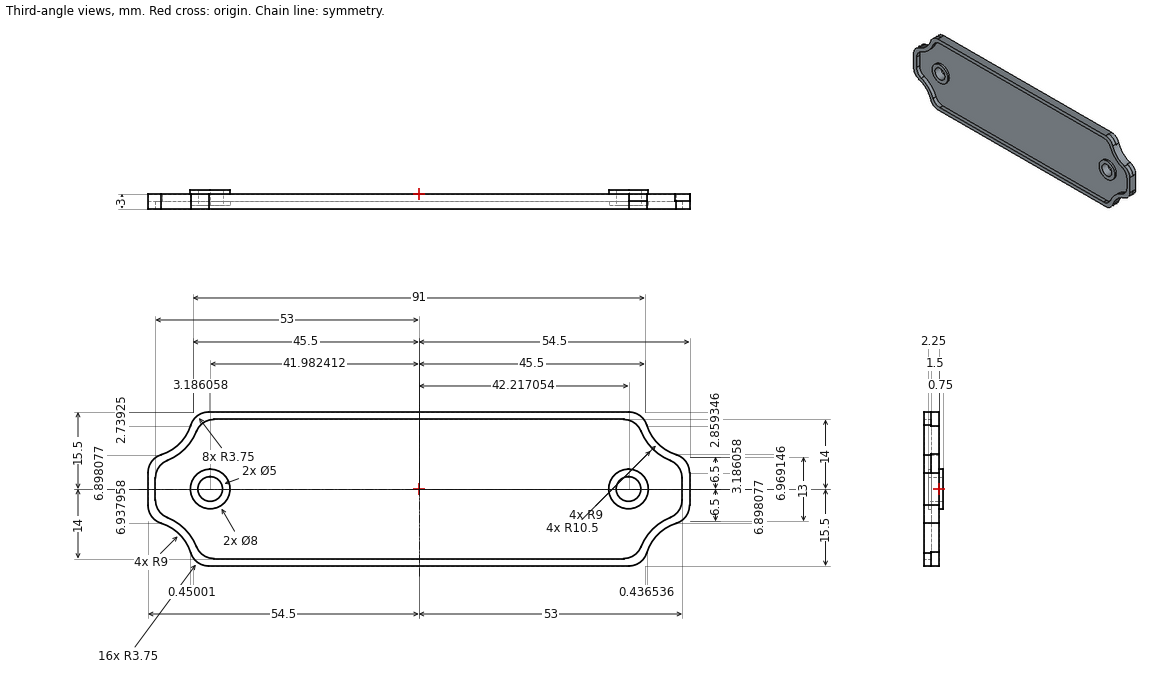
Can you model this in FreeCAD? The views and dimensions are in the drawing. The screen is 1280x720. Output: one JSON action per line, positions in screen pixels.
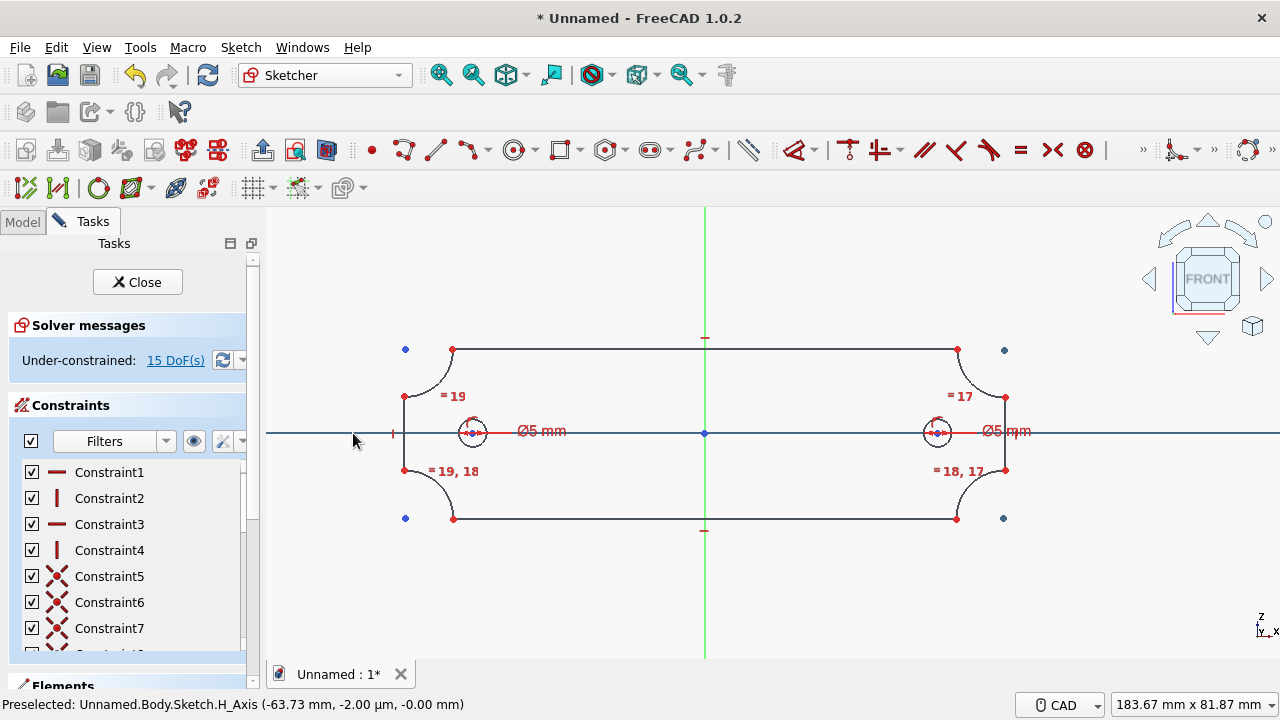
{"action": "left_click", "coordinate": [1054, 150]}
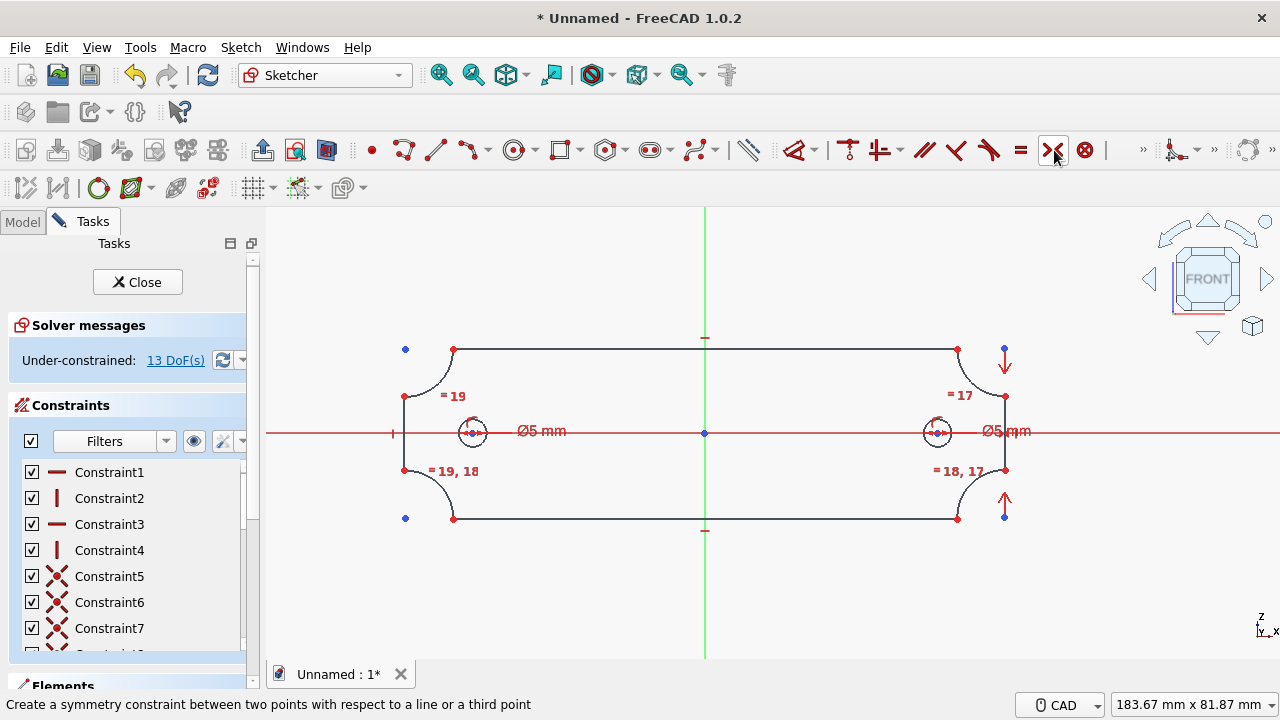
{"action": "left_click", "coordinate": [1005, 517]}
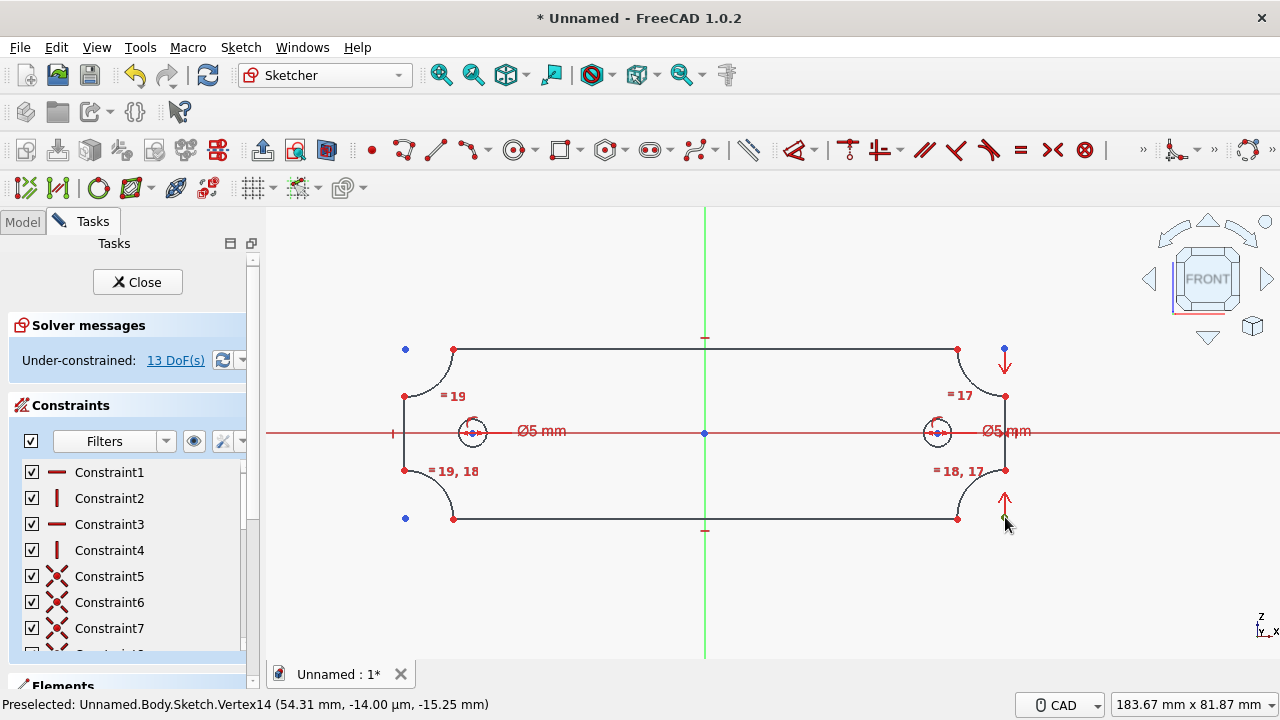
{"action": "left_click", "coordinate": [406, 518]}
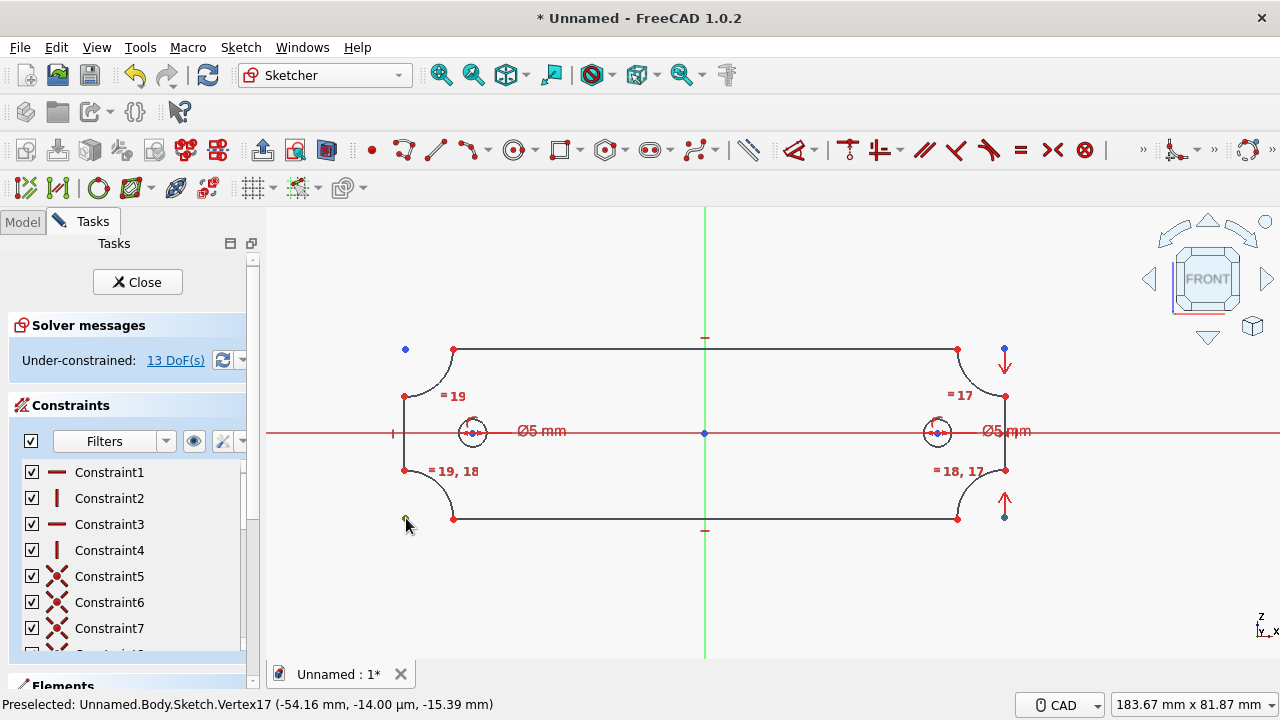
{"action": "left_click", "coordinate": [705, 603]}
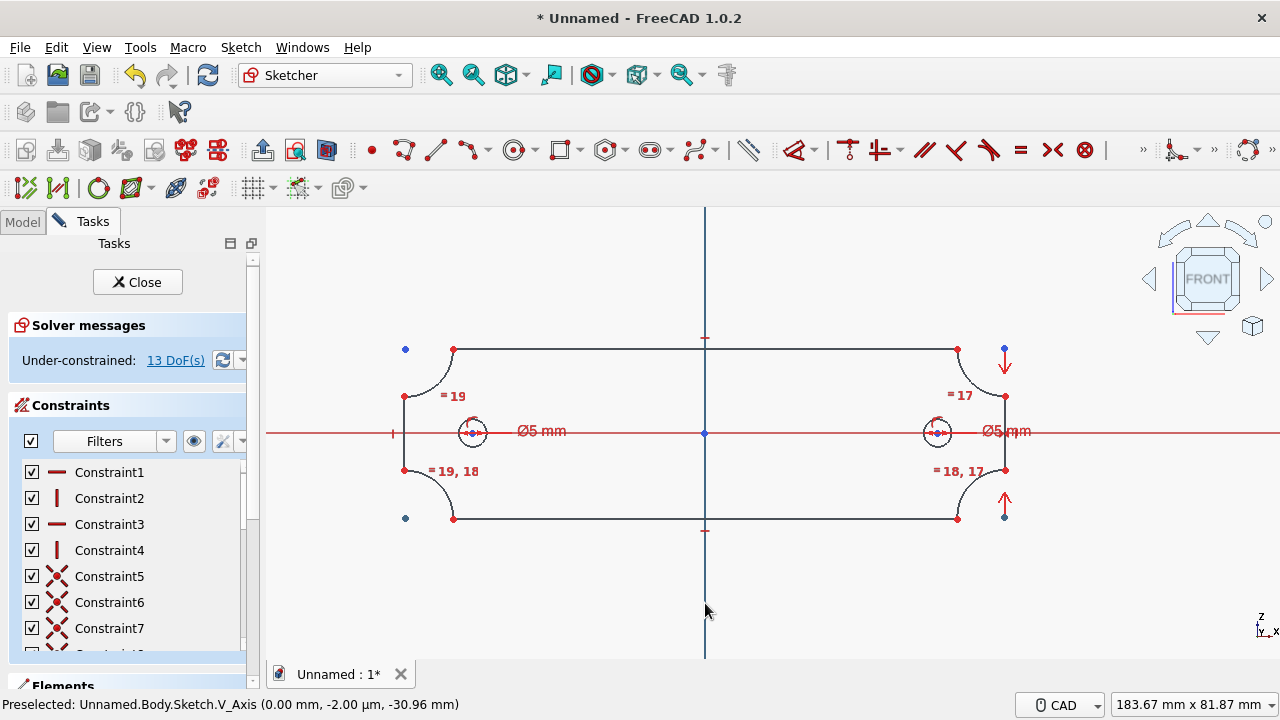
{"action": "left_click", "coordinate": [1054, 150]}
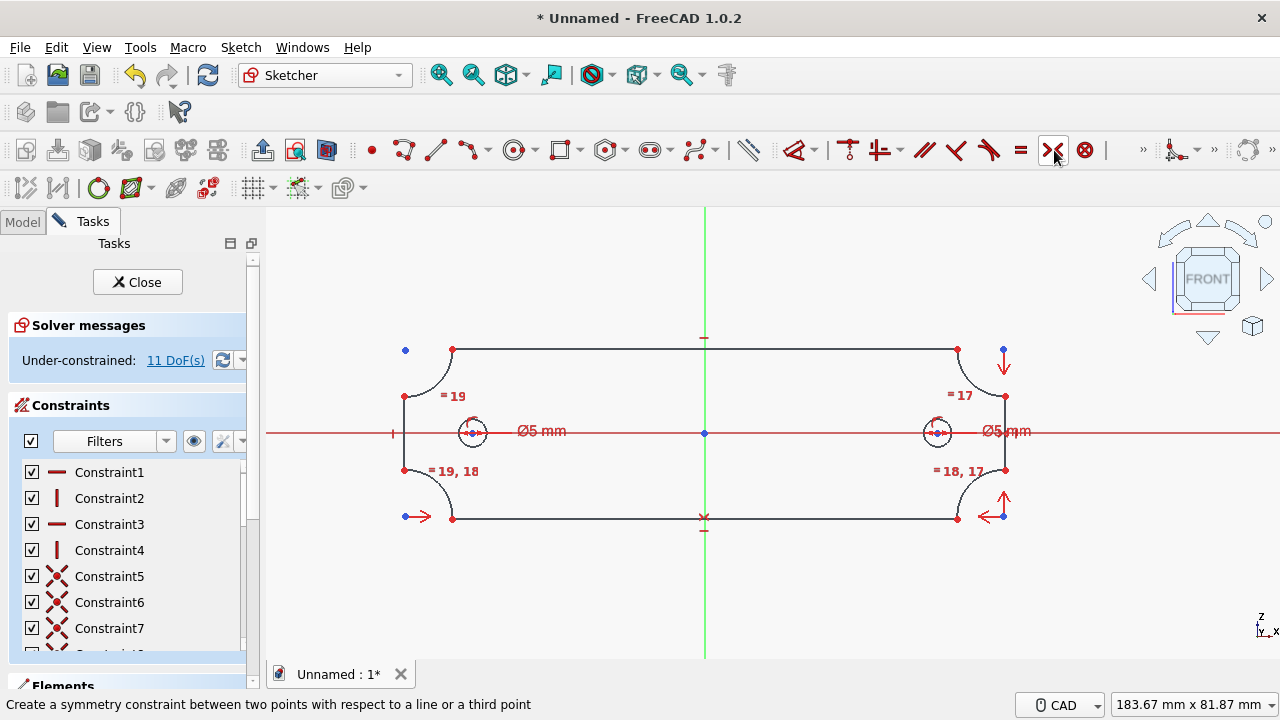
{"action": "left_click", "coordinate": [1004, 350]}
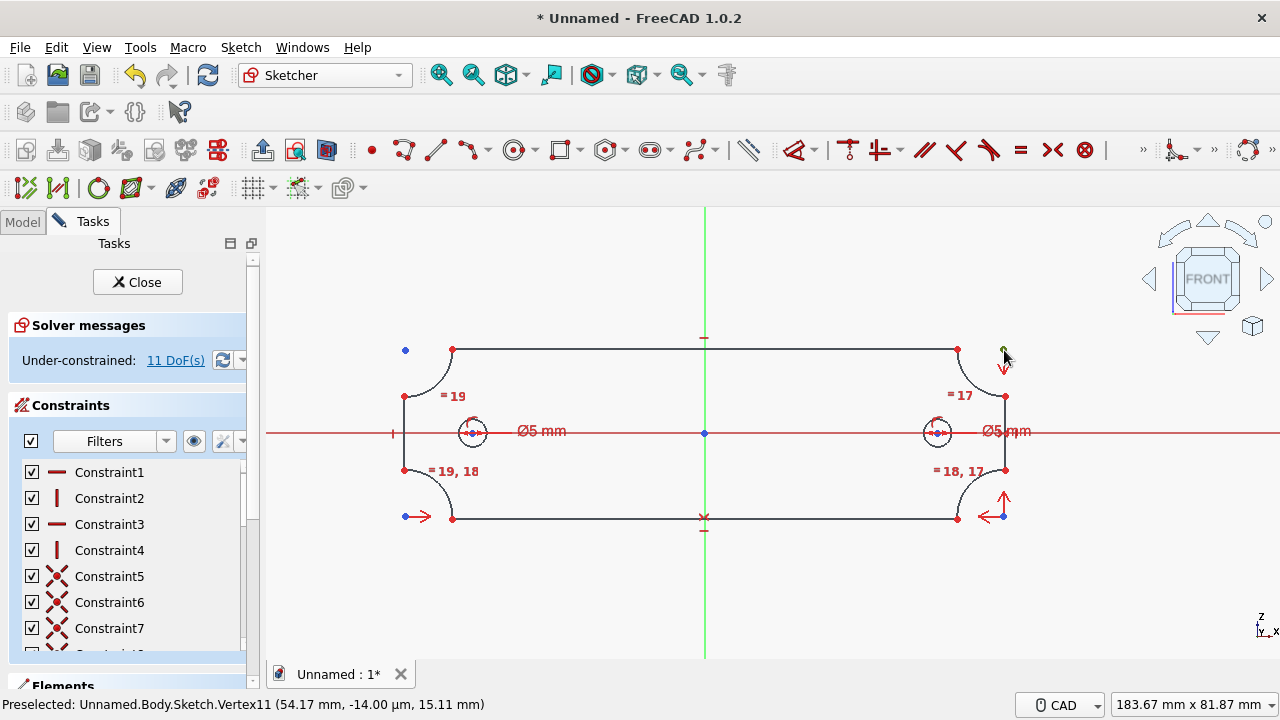
{"action": "left_click", "coordinate": [406, 350]}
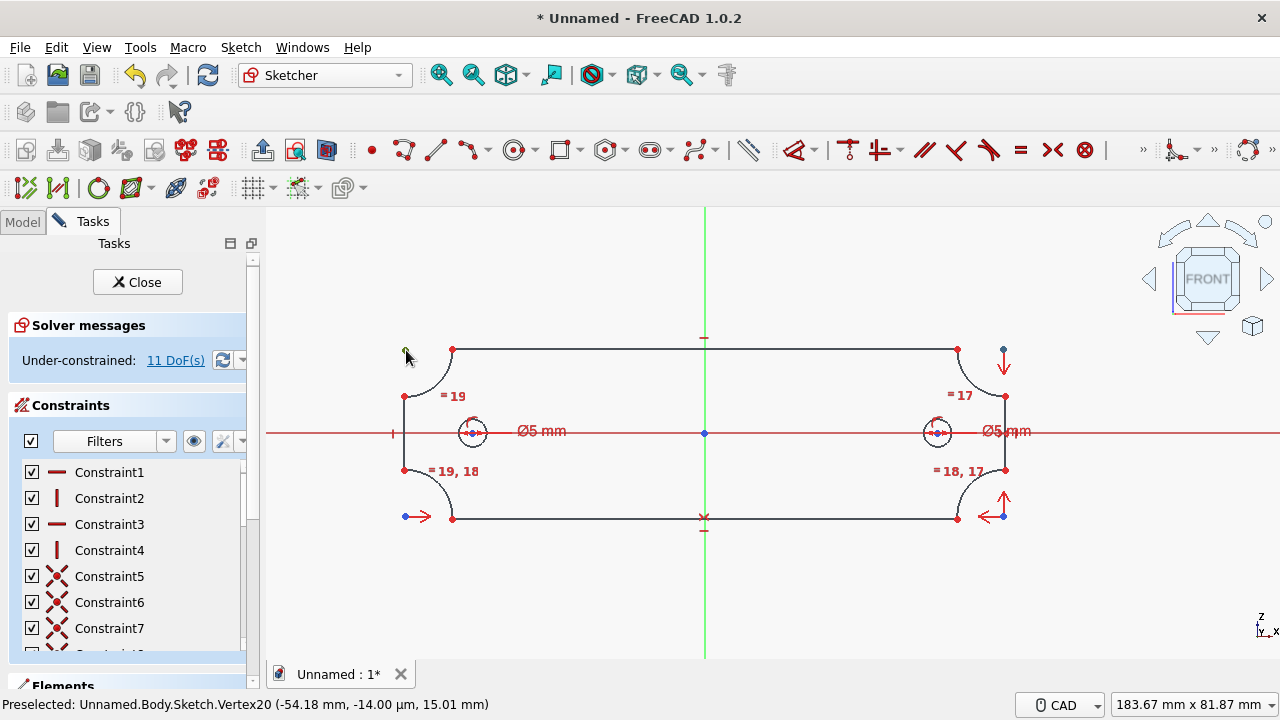
{"action": "left_click", "coordinate": [705, 603]}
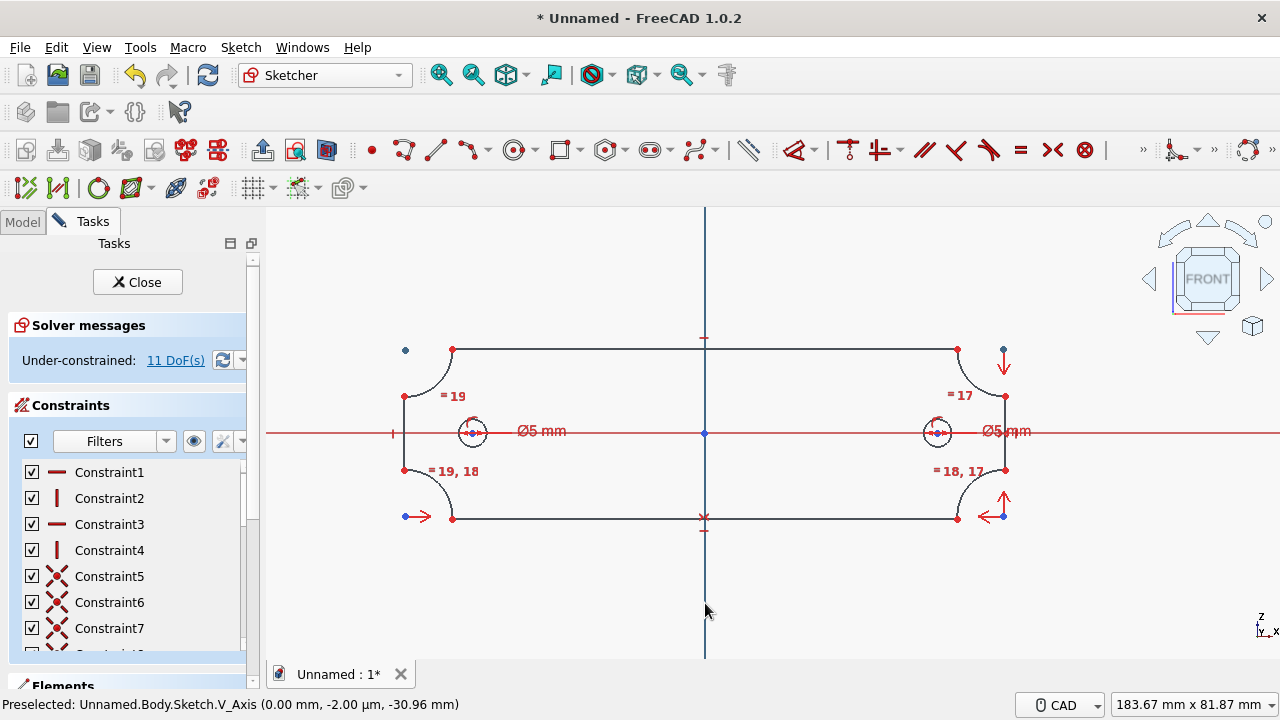
{"action": "left_click", "coordinate": [1054, 150]}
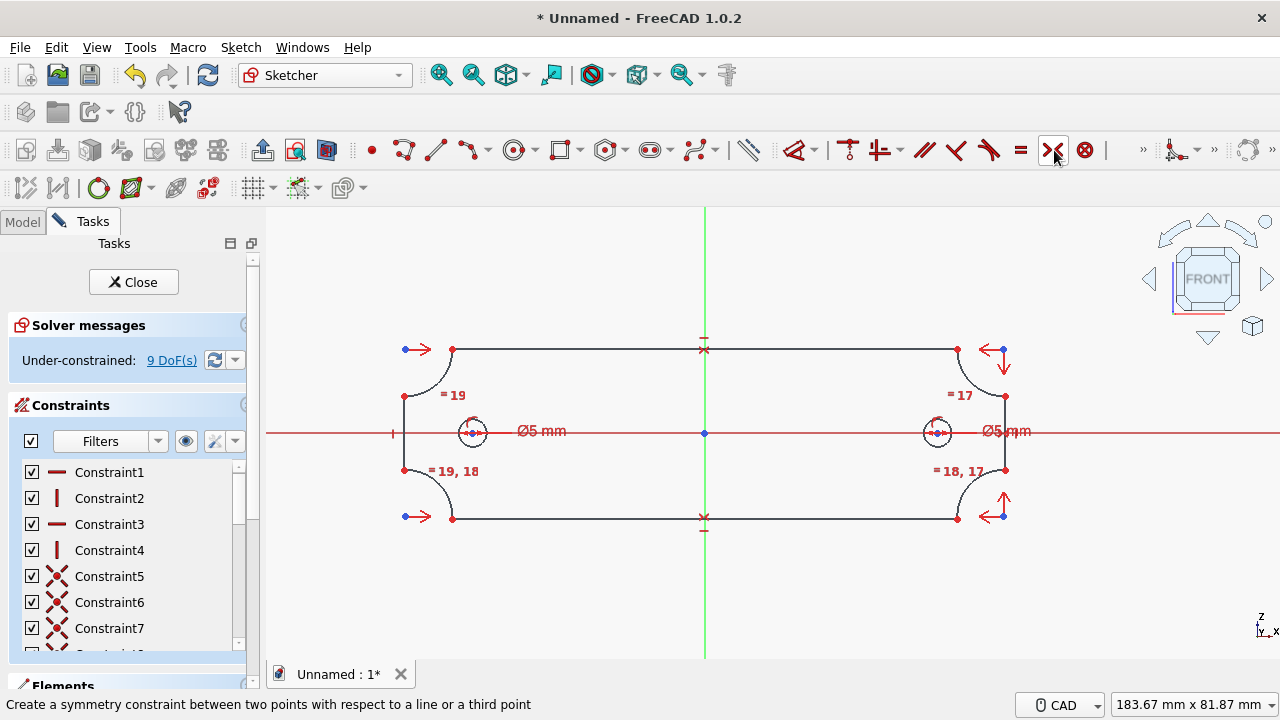
{"action": "left_click", "coordinate": [794, 150]}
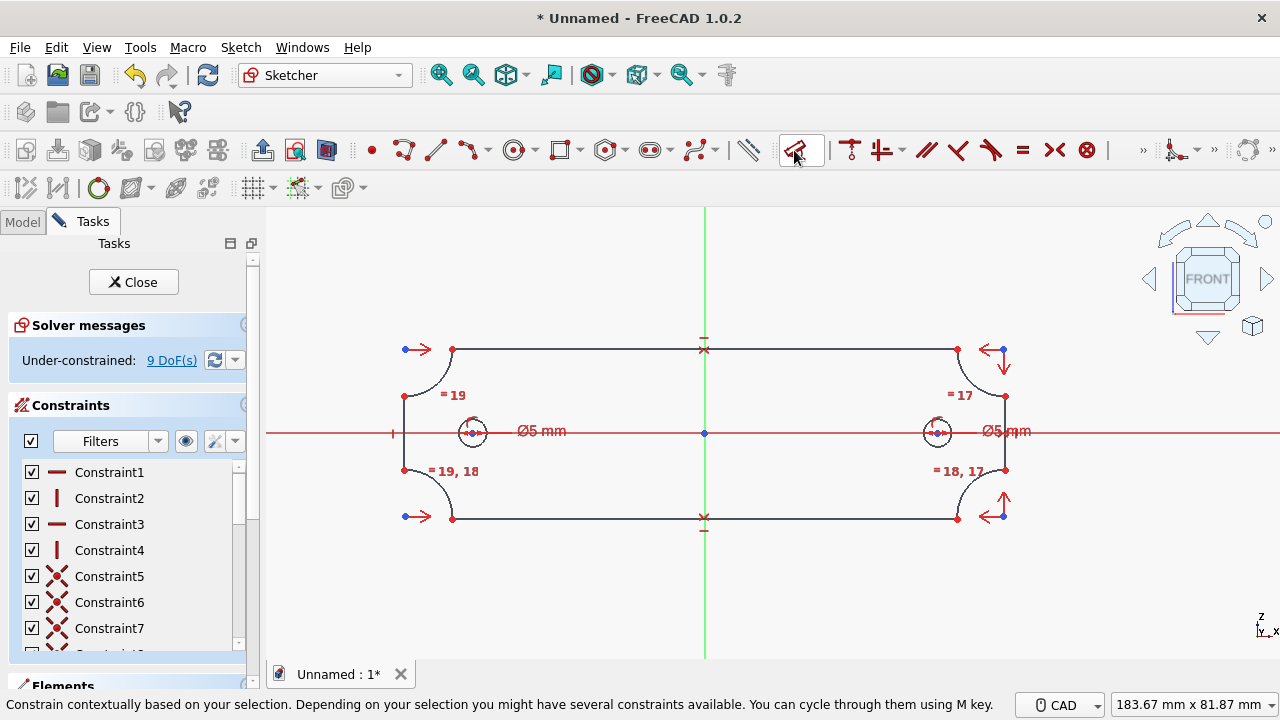
{"action": "left_click", "coordinate": [962, 371]}
{"action": "left_click", "coordinate": [933, 386]}